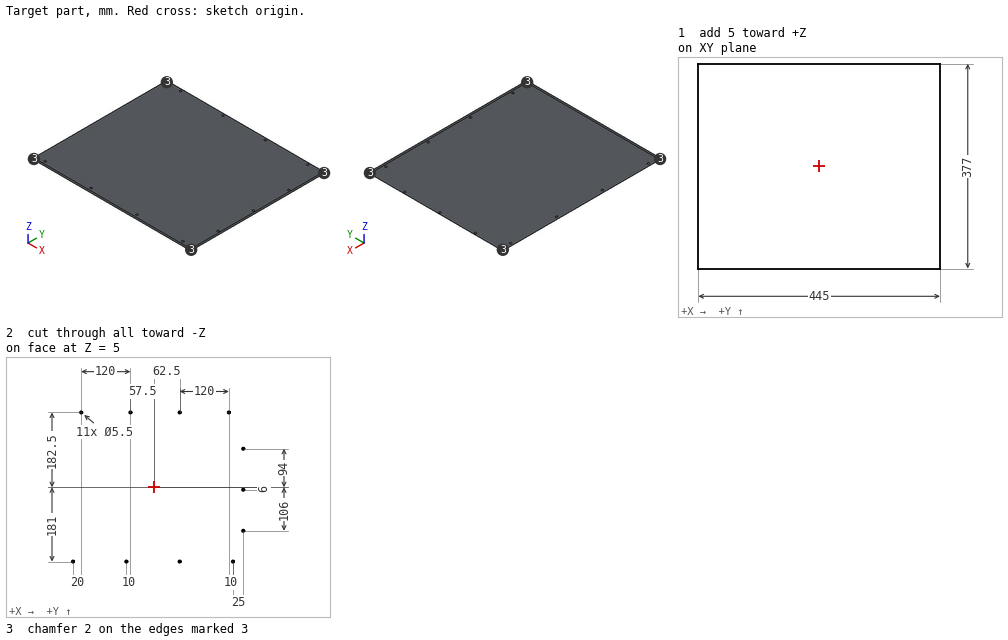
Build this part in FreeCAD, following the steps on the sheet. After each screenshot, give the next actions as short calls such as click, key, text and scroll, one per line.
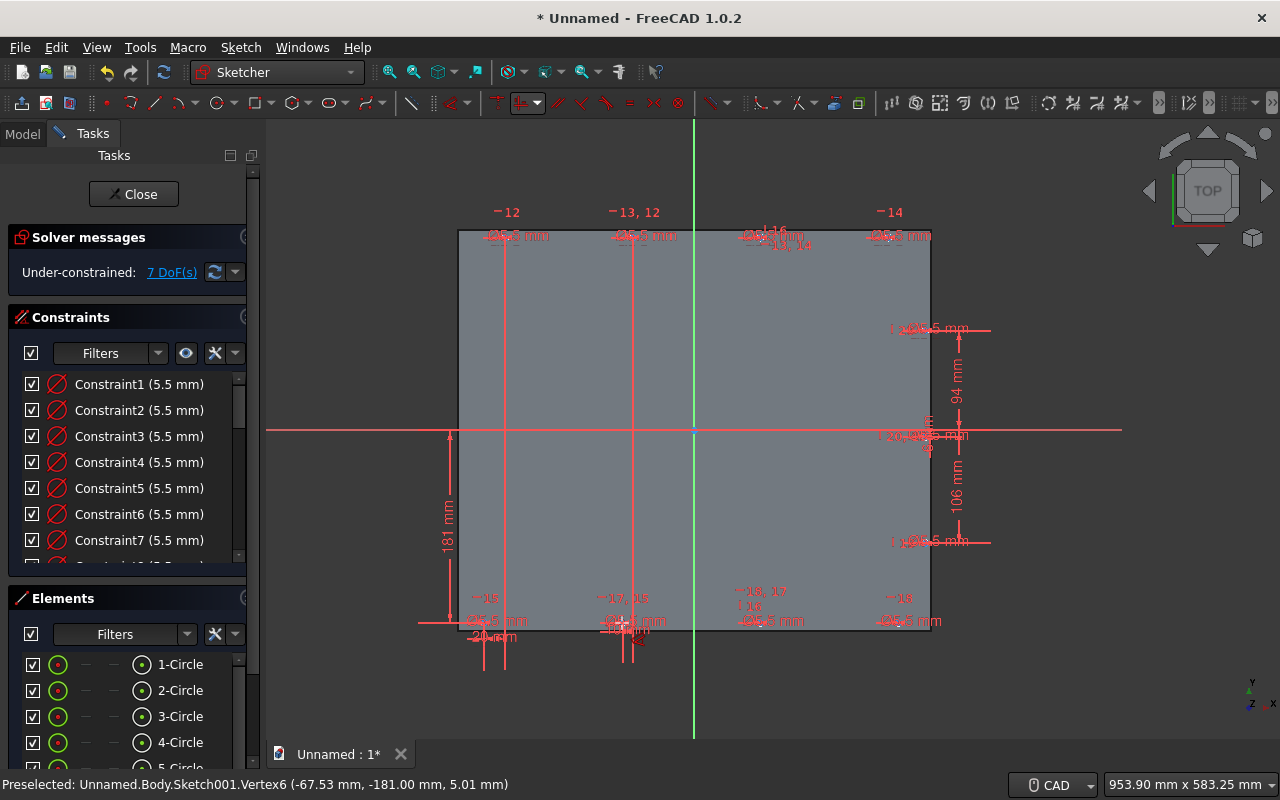
scroll(888, 238, up, 7)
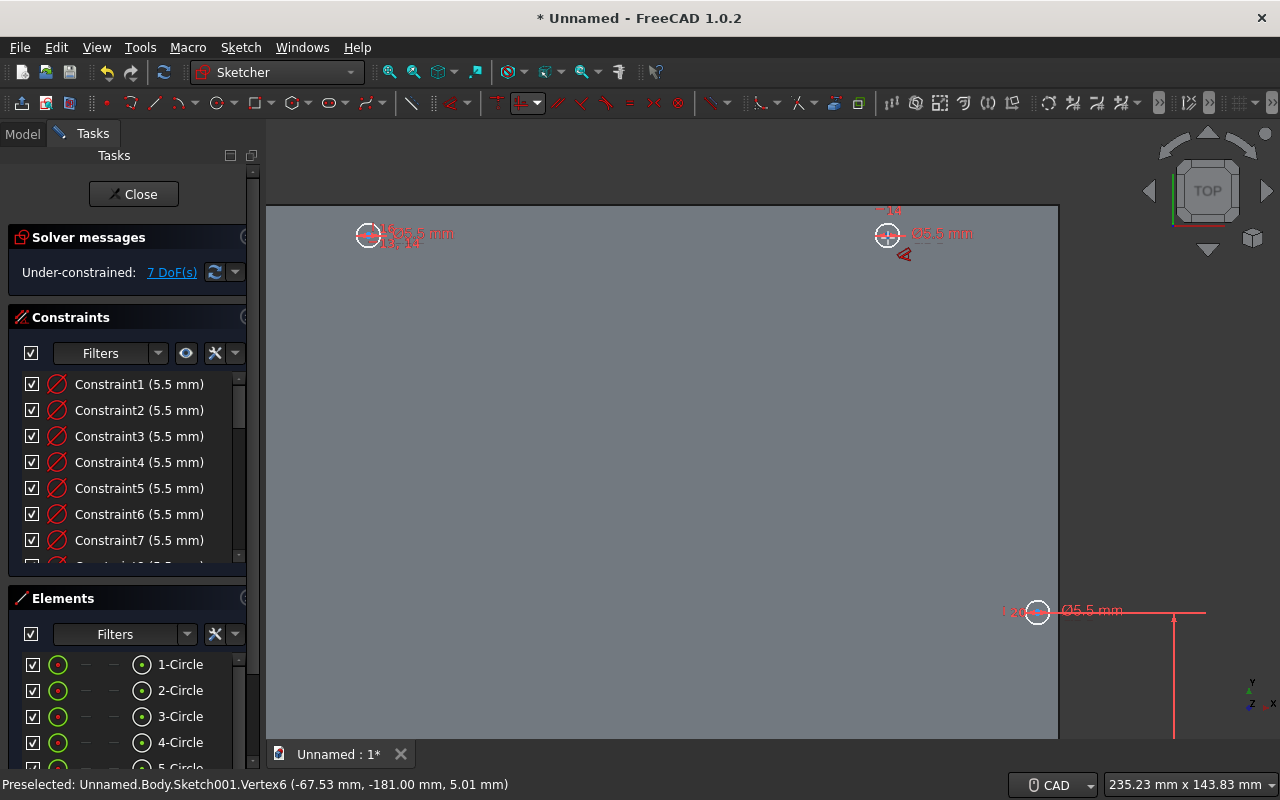
click(888, 236)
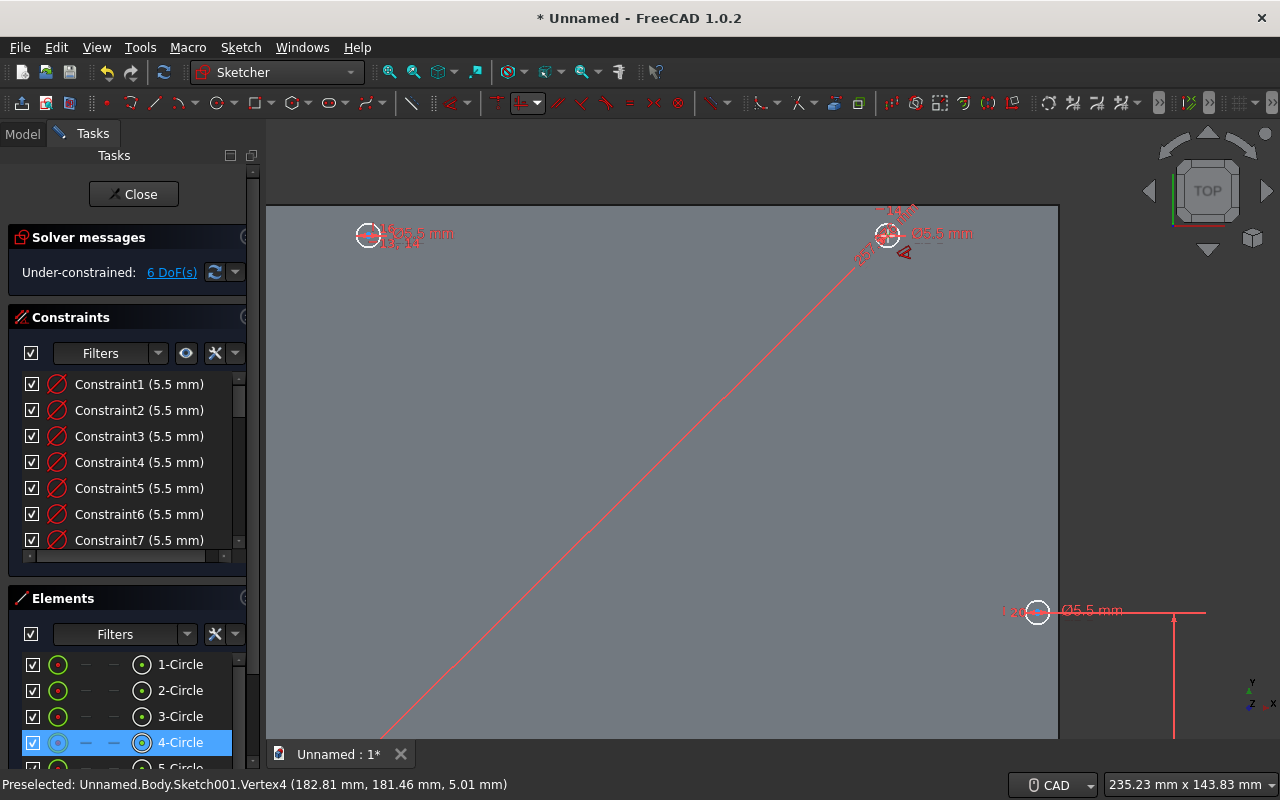
scroll(888, 237, down, 7)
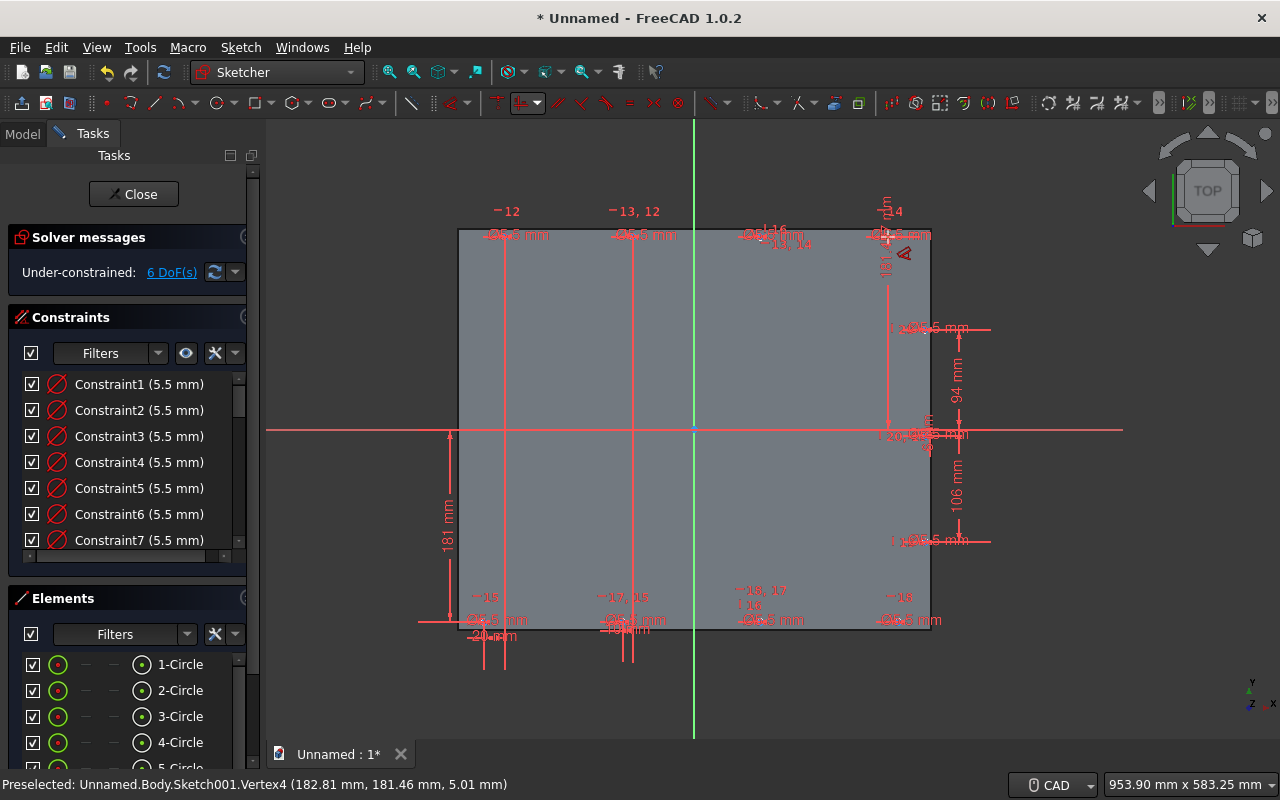
scroll(898, 622, up, 7)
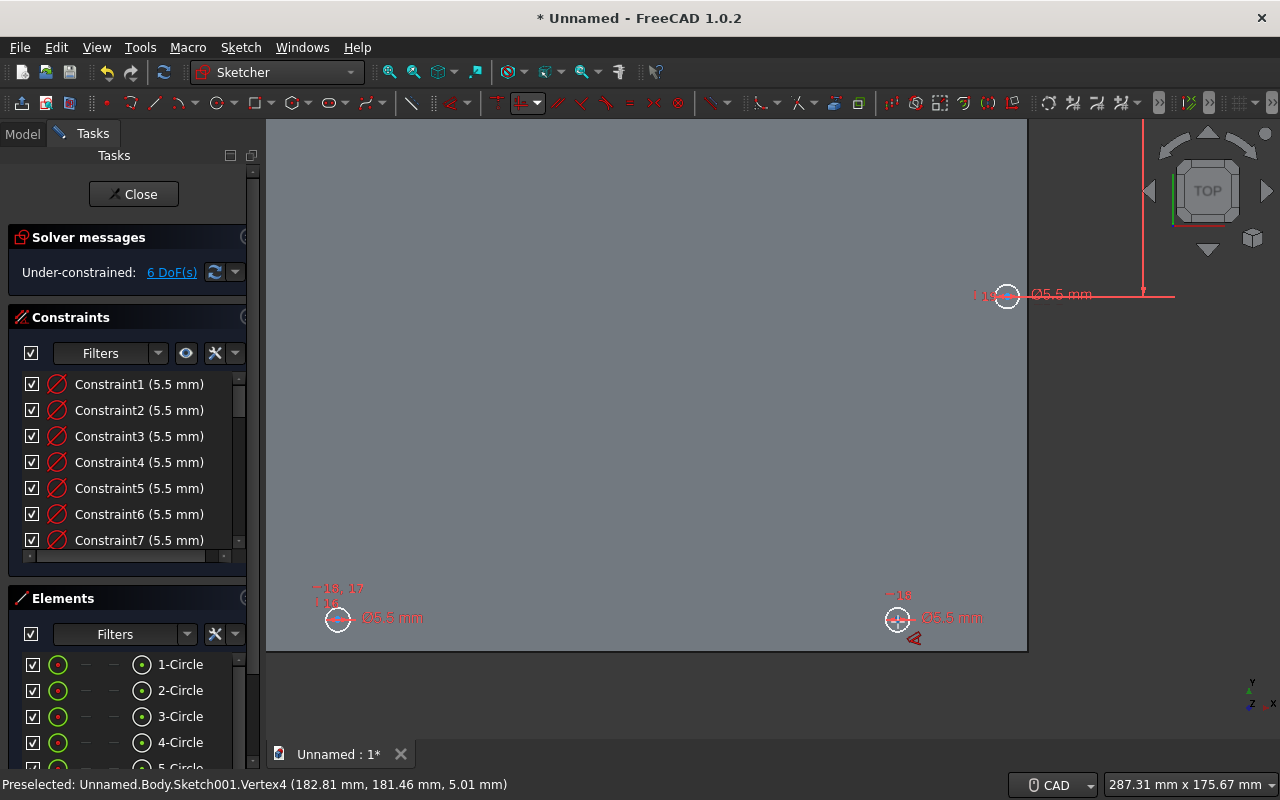
click(898, 620)
click(877, 654)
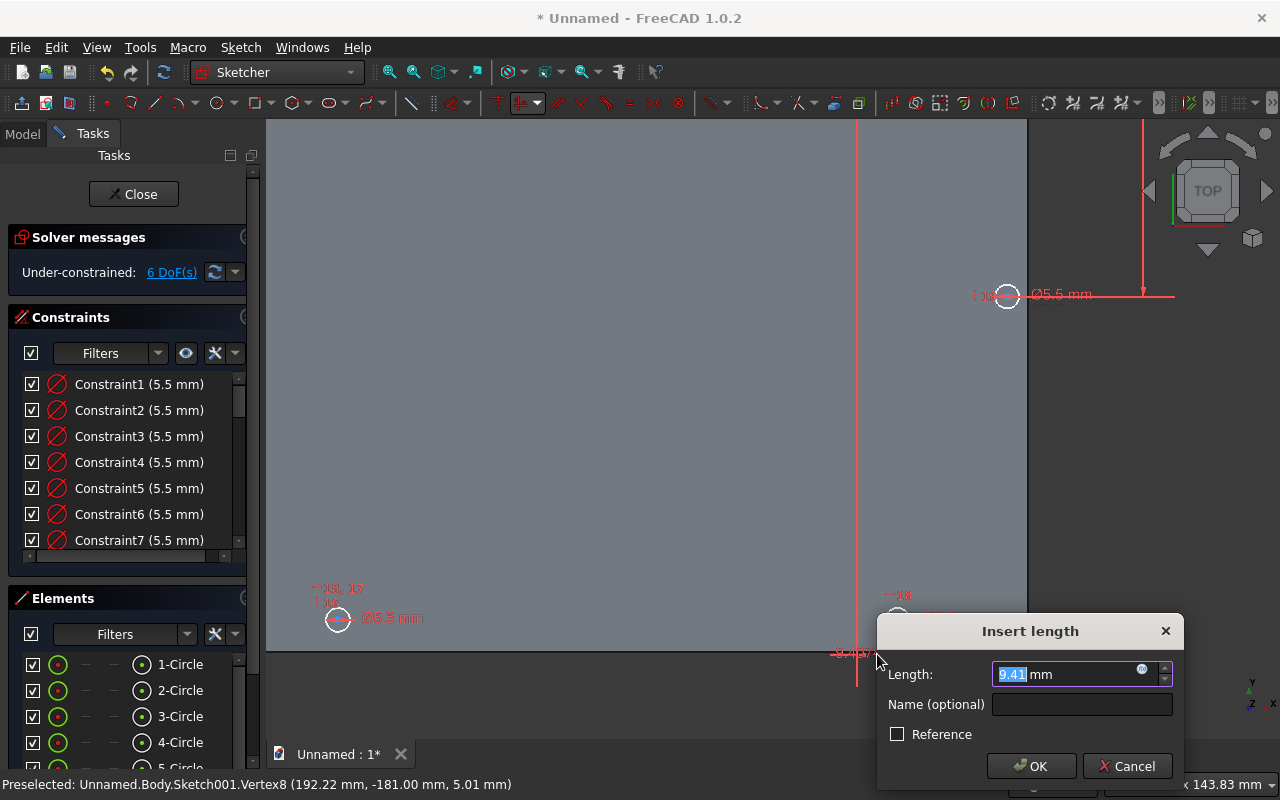
text(10)
key(Return)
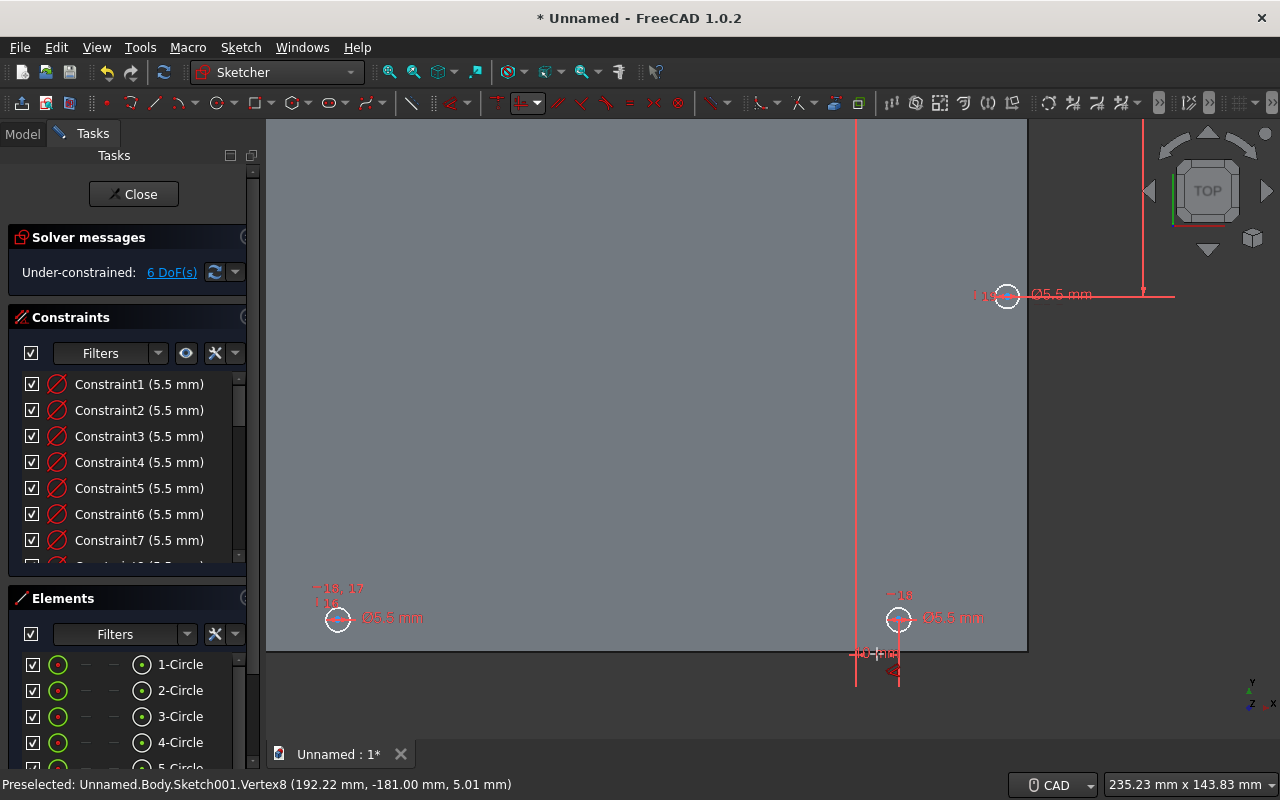
click(899, 620)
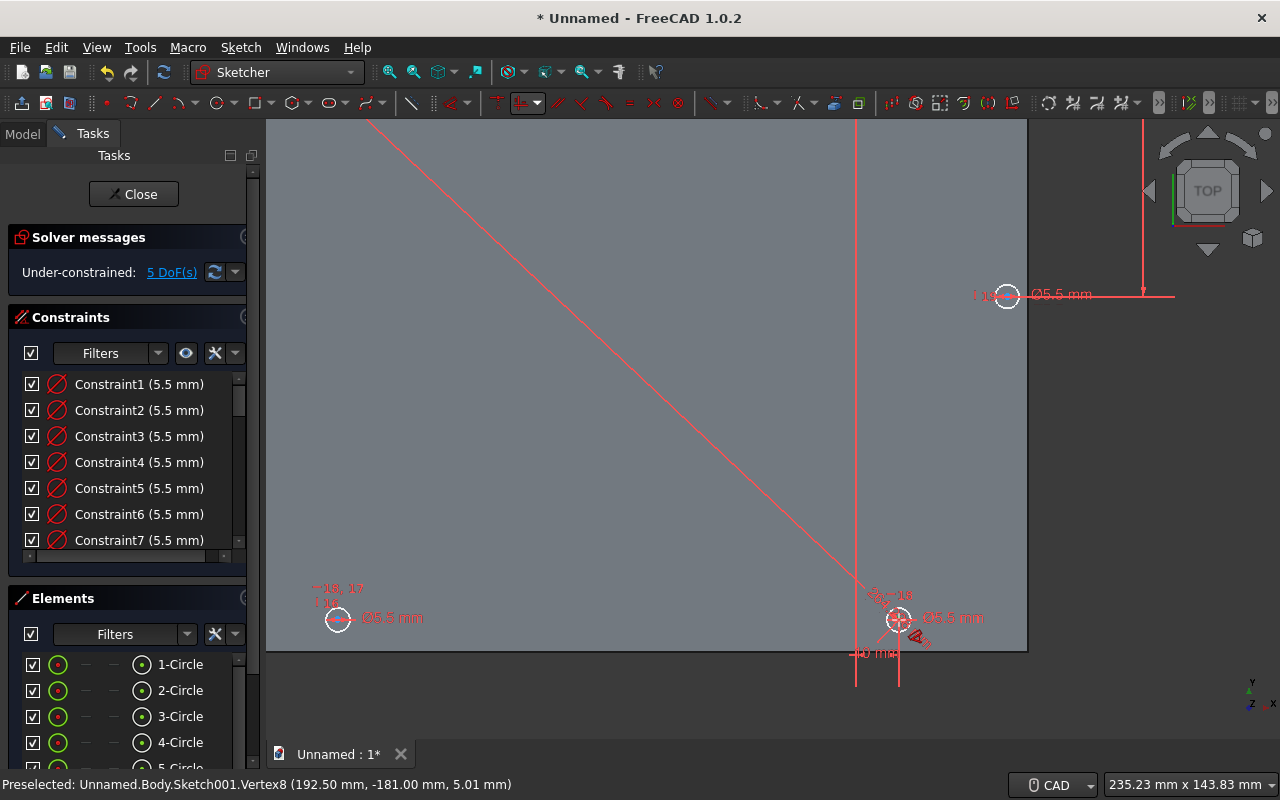
click(1007, 297)
click(953, 654)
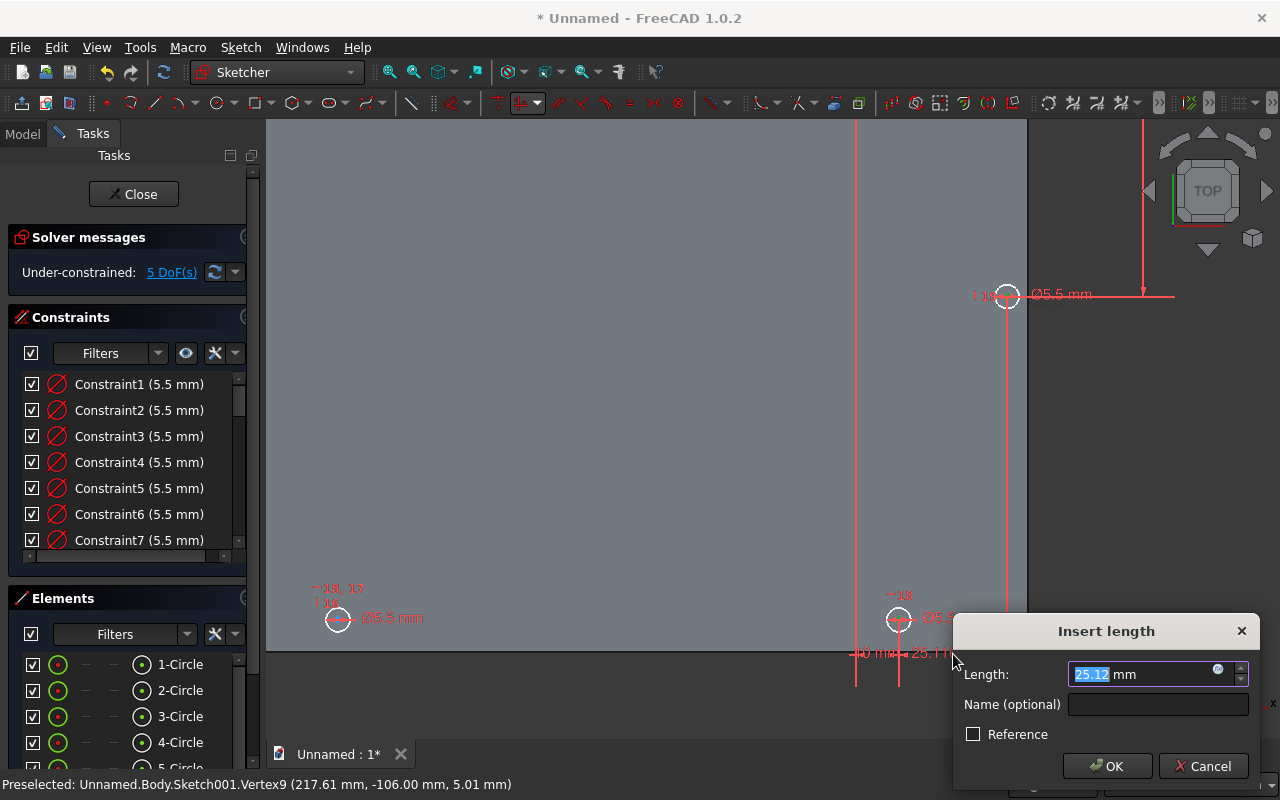
text(25)
key(Return)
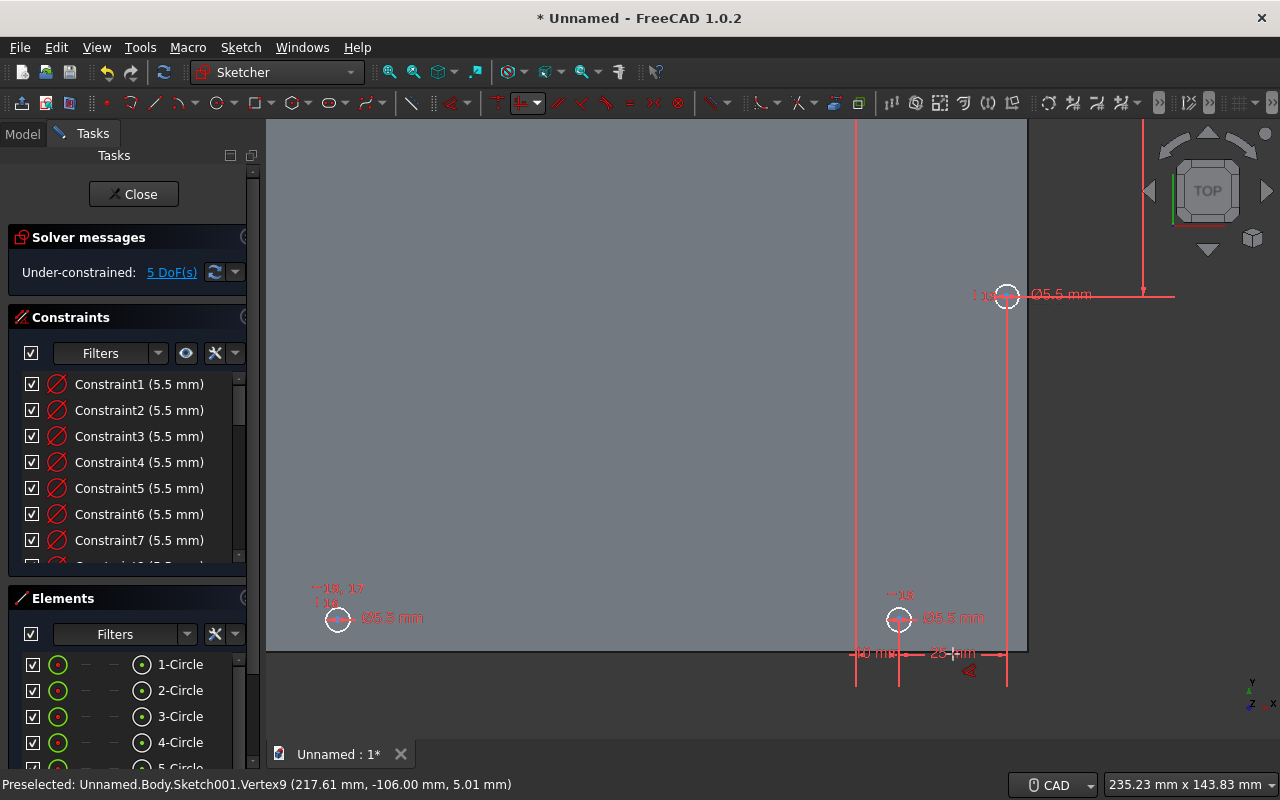
scroll(898, 623, down, 7)